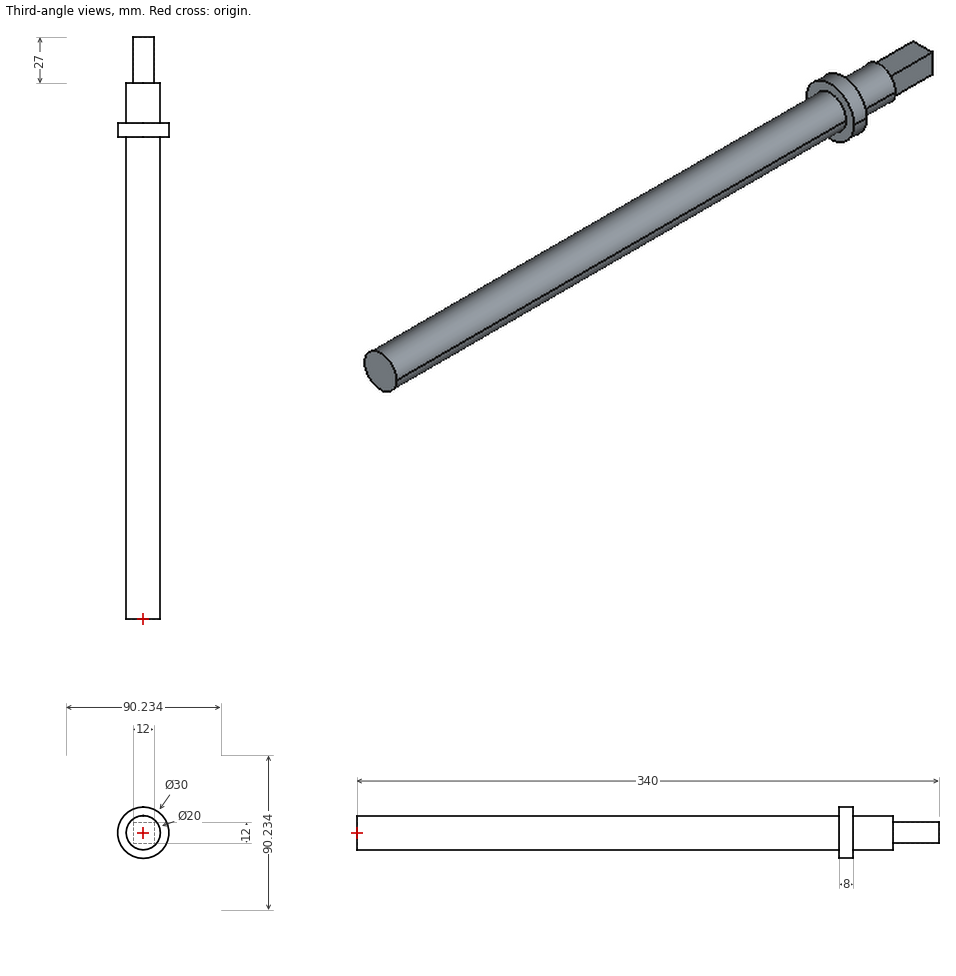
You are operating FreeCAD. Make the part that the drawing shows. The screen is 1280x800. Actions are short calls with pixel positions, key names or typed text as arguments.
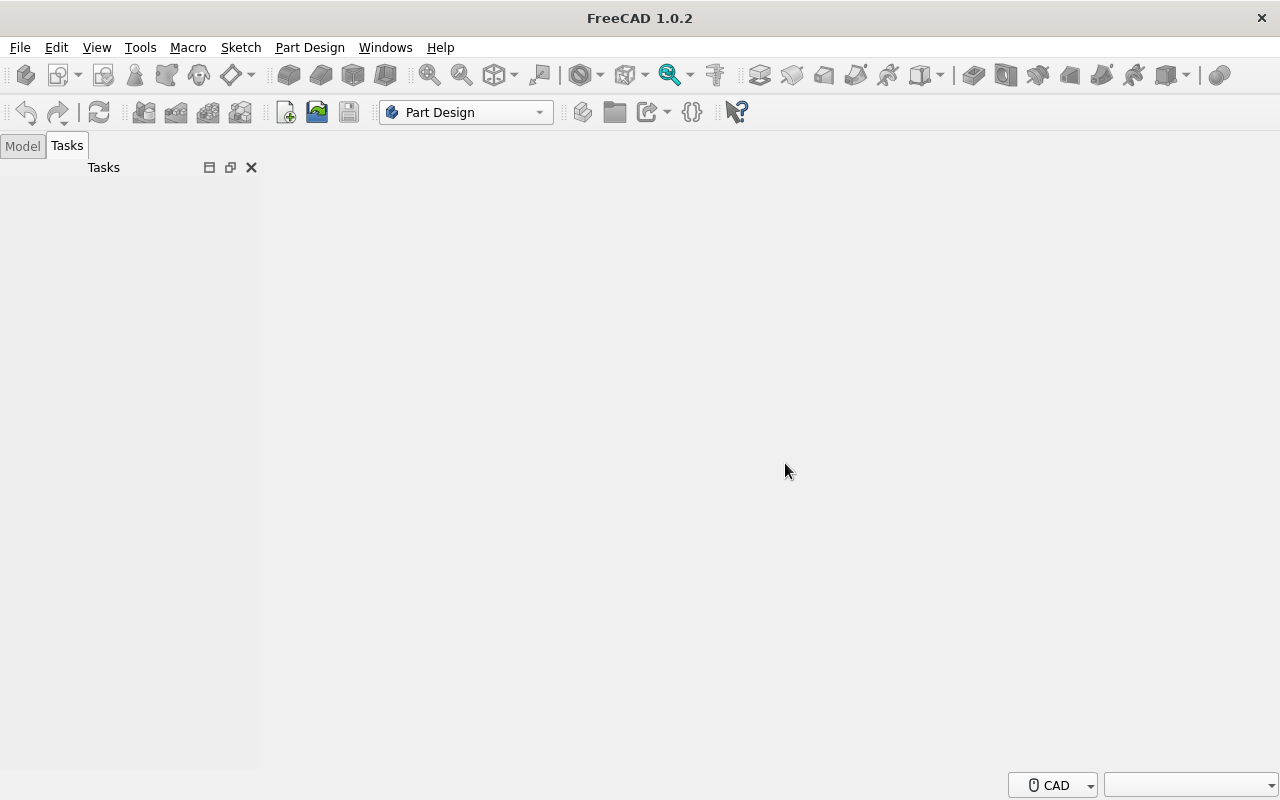
click(286, 112)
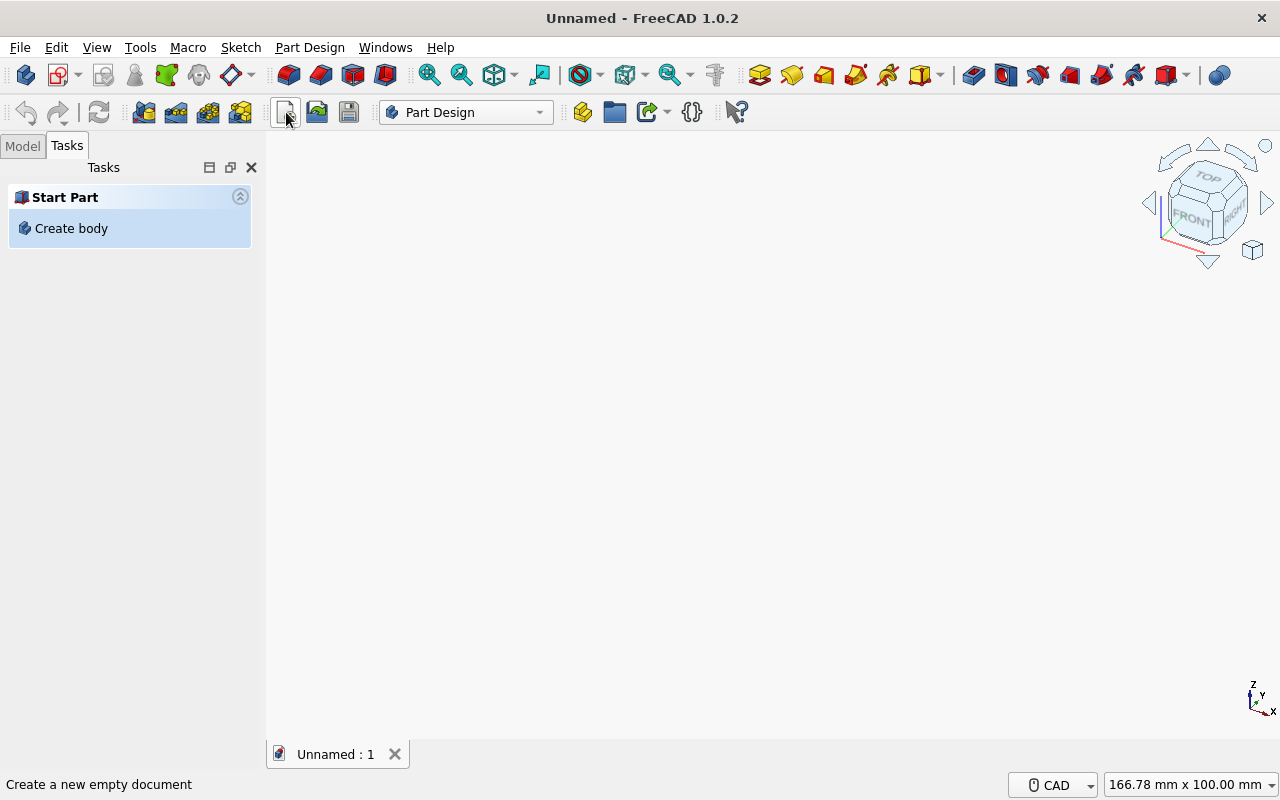
click(58, 76)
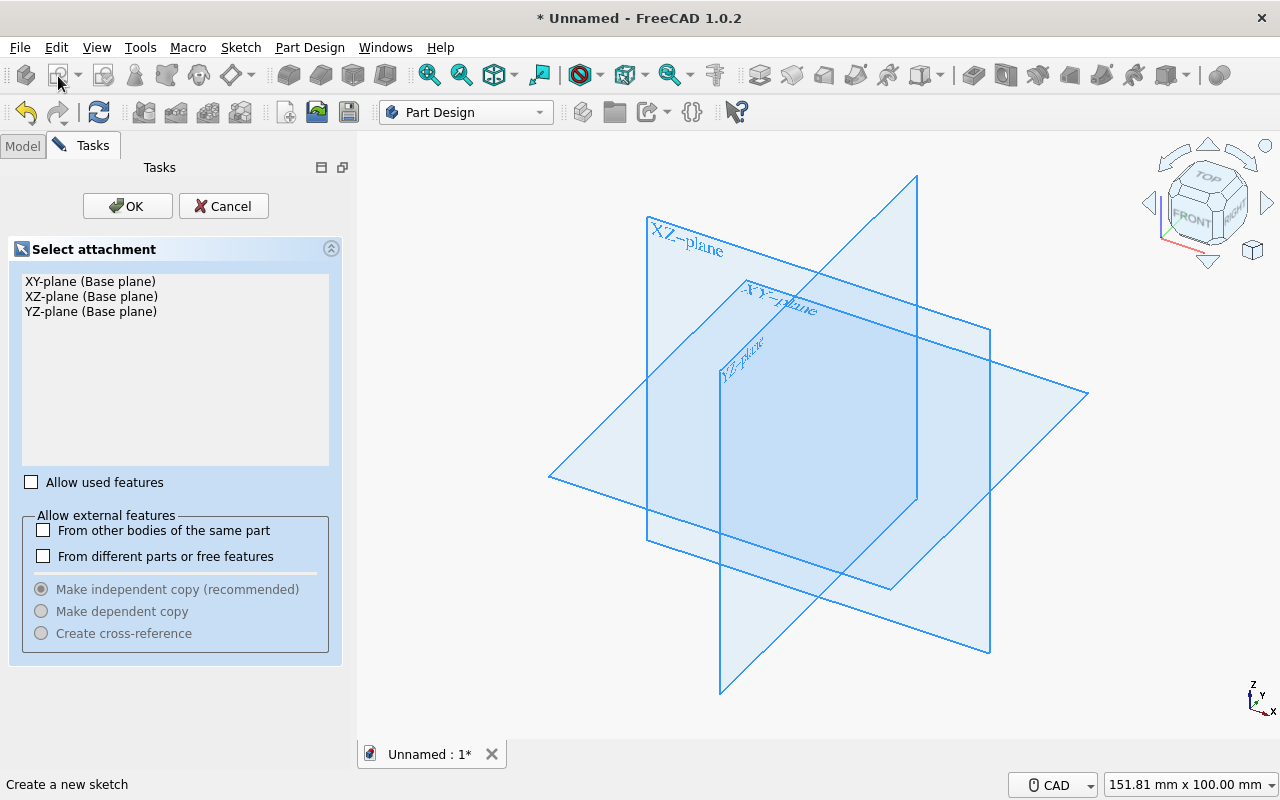
click(82, 296)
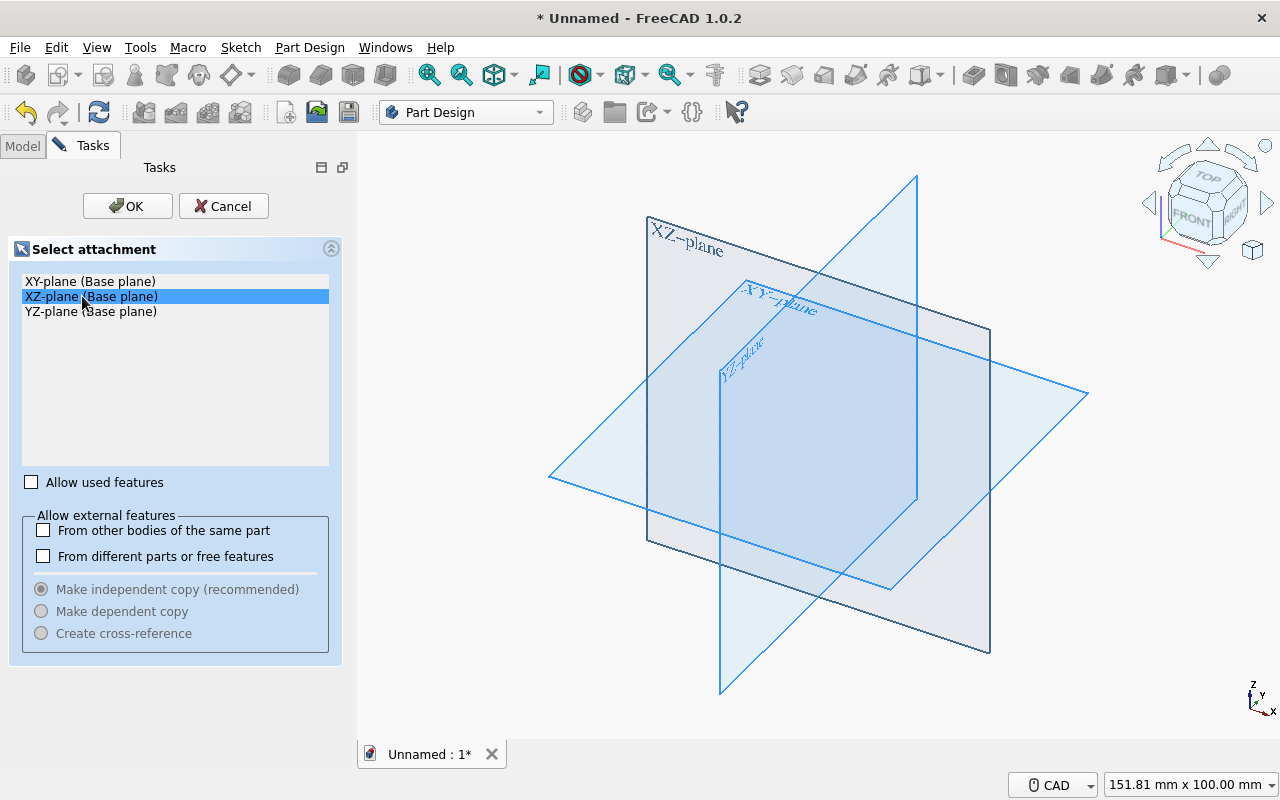
click(128, 206)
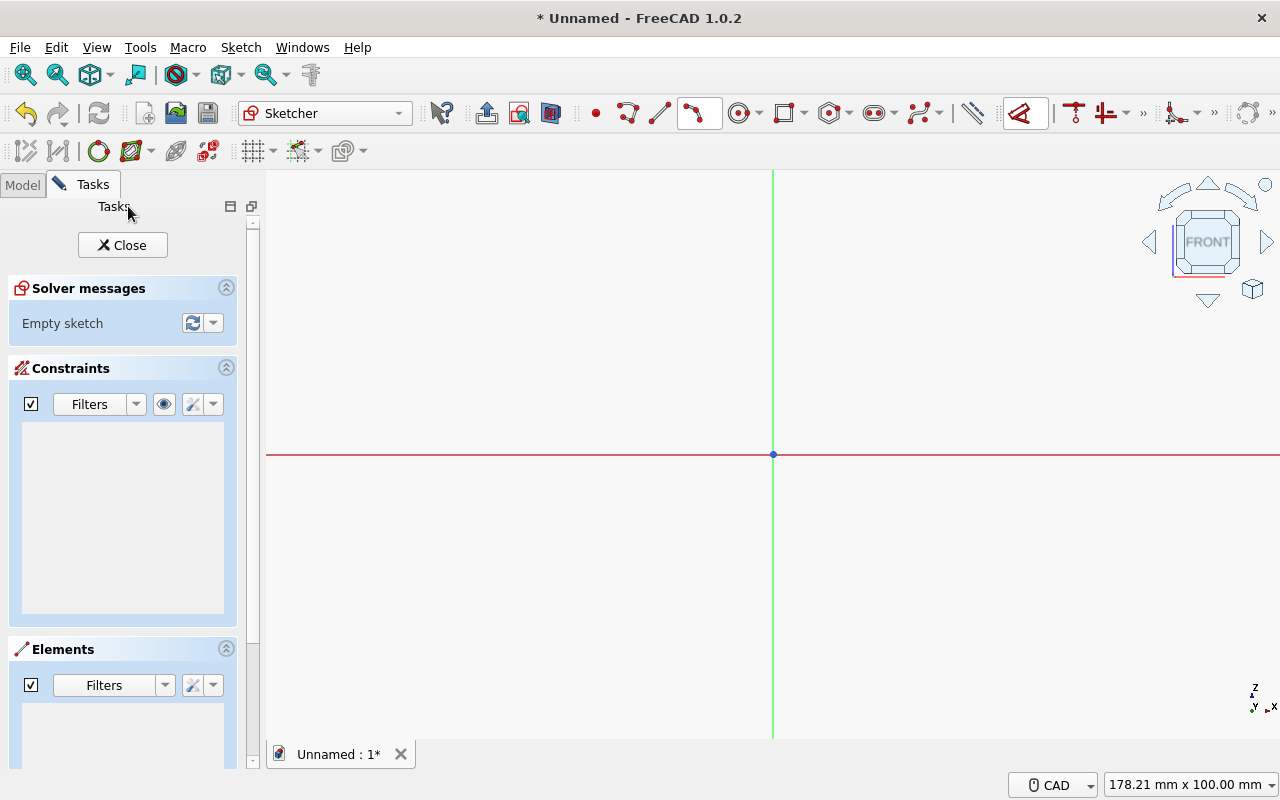
scroll(803, 455, up, 6)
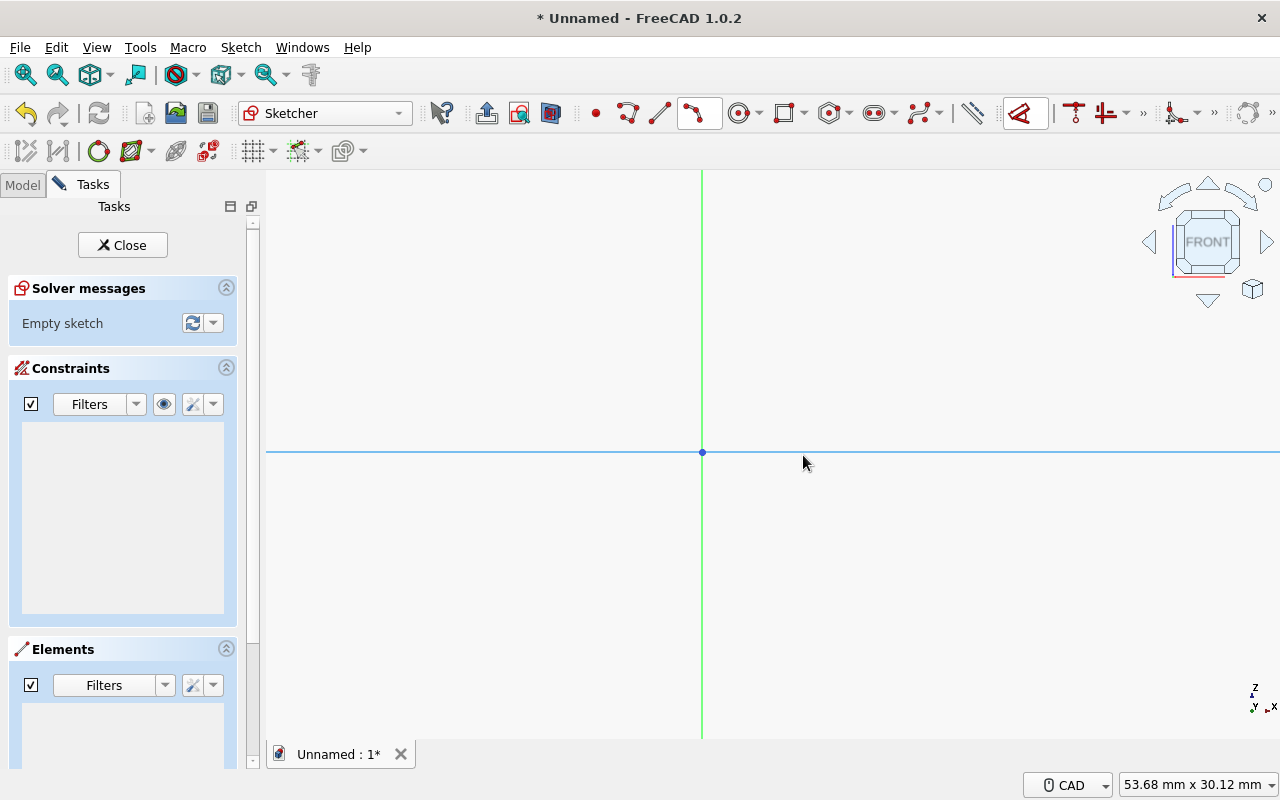
click(740, 114)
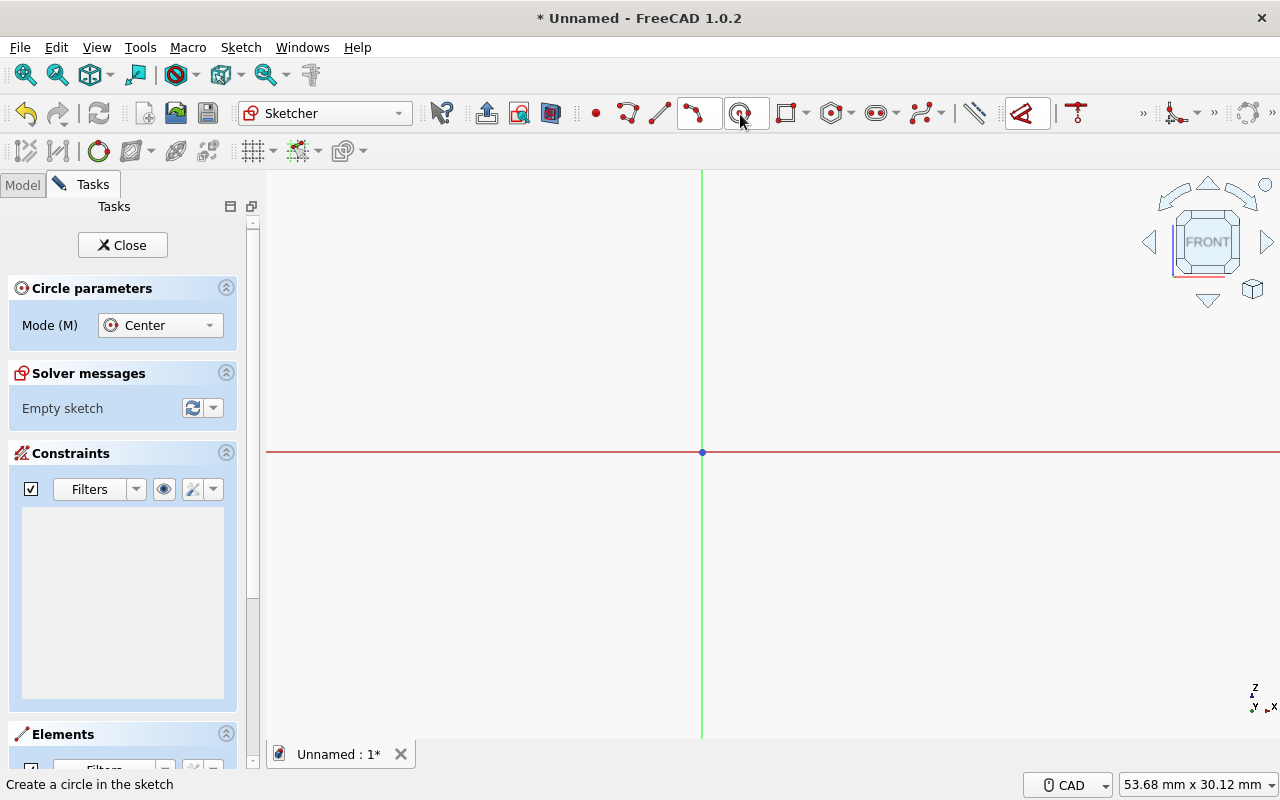
click(702, 452)
move(836, 319)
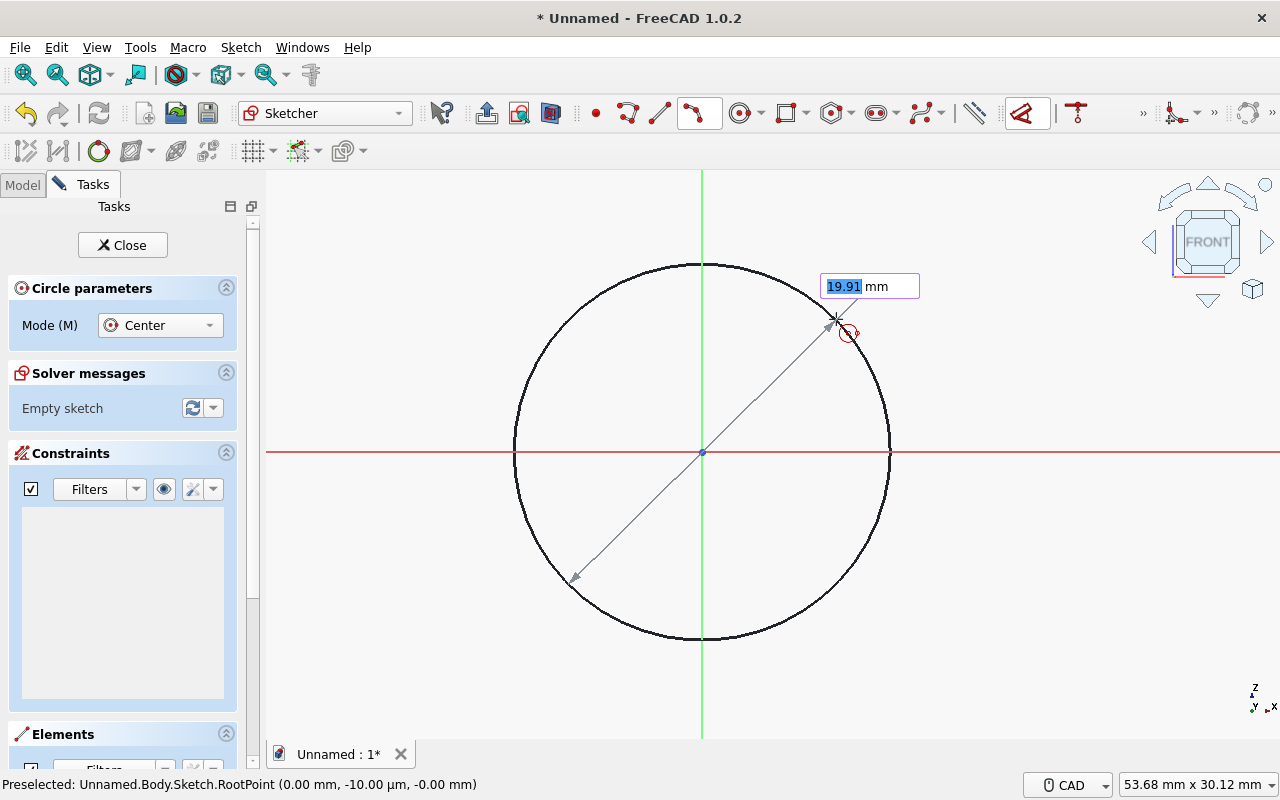
text(20)
key(Return)
key(Escape)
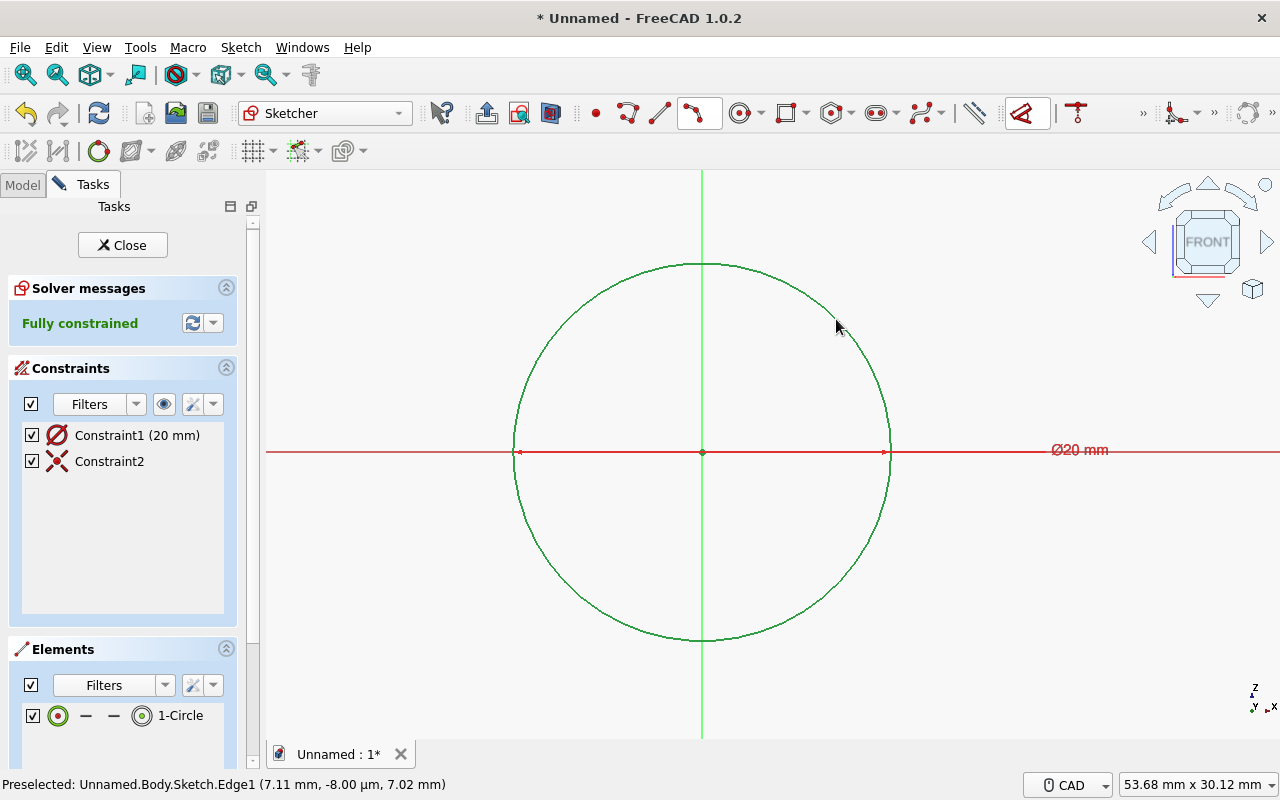
click(123, 245)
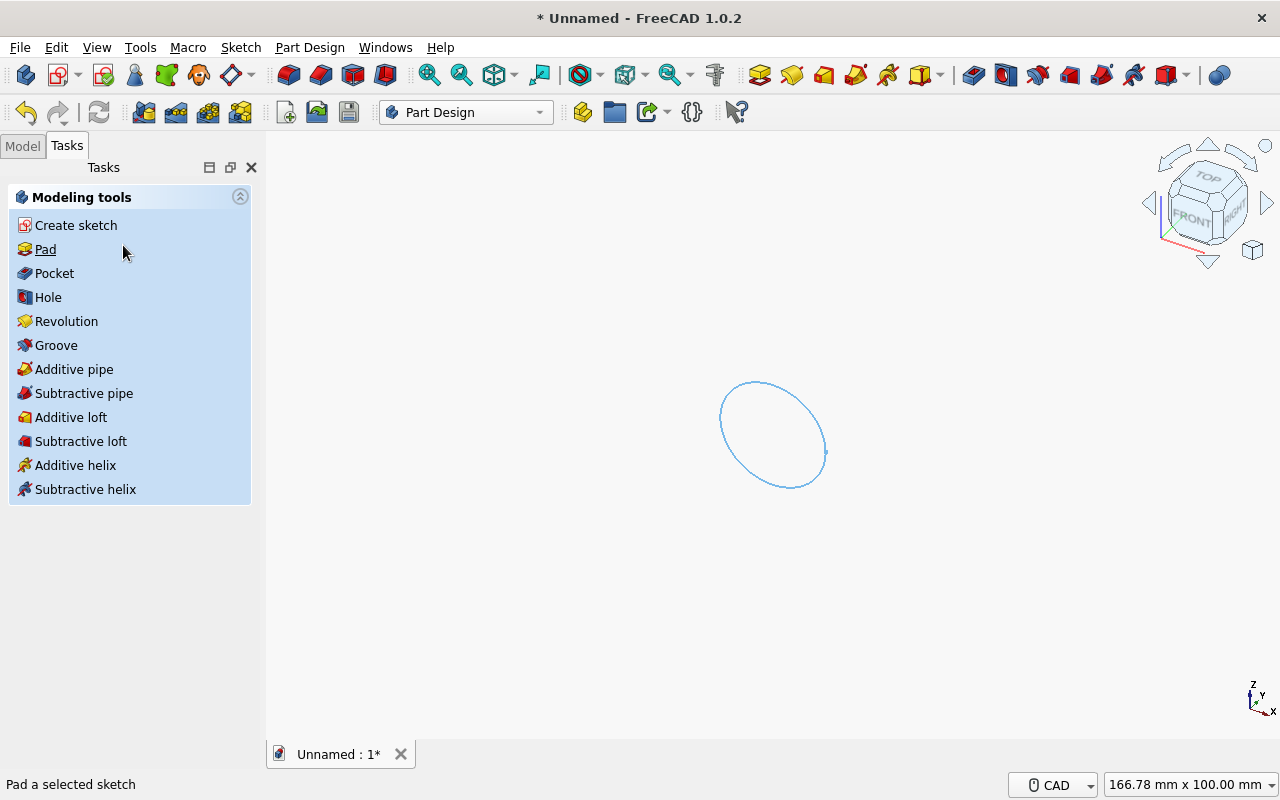
click(760, 76)